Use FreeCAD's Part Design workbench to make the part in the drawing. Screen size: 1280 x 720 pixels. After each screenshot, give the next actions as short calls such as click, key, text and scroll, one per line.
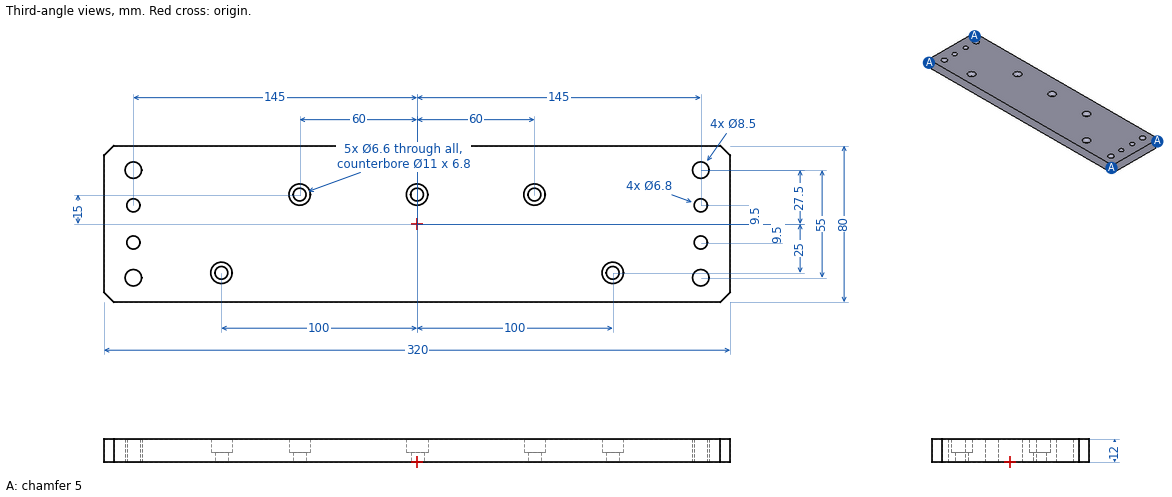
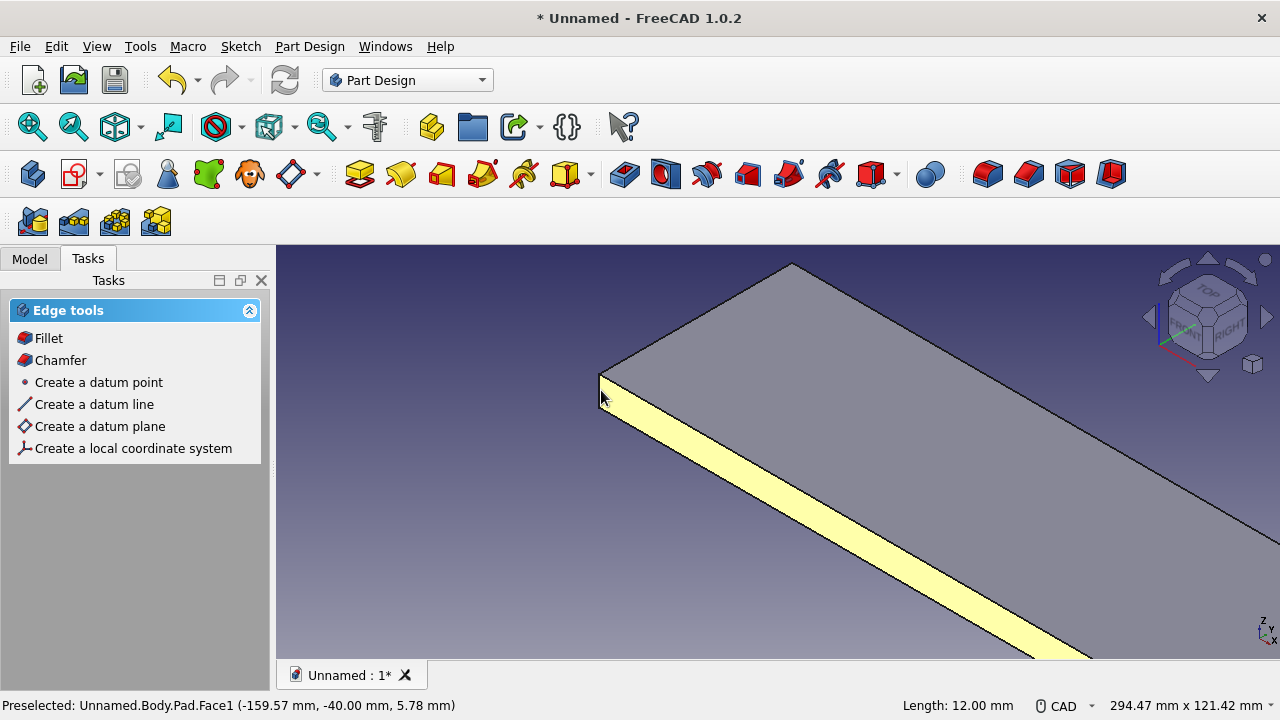
click(33, 128)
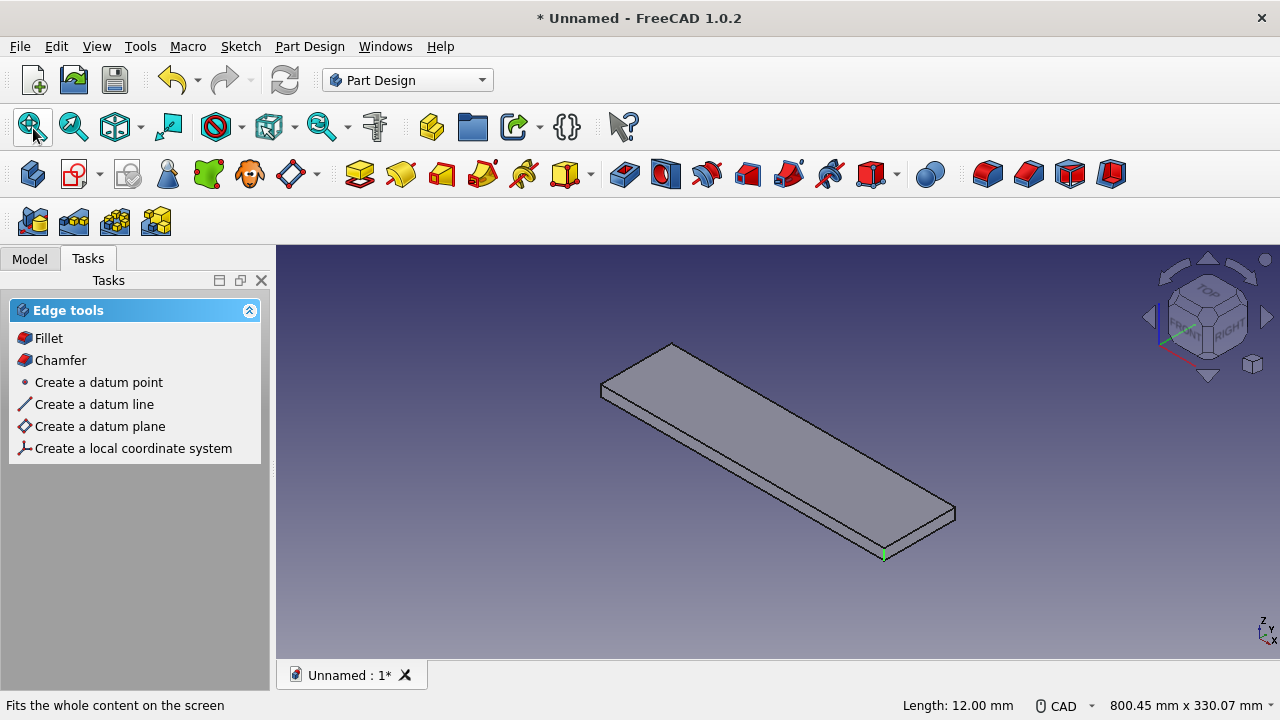
key(2)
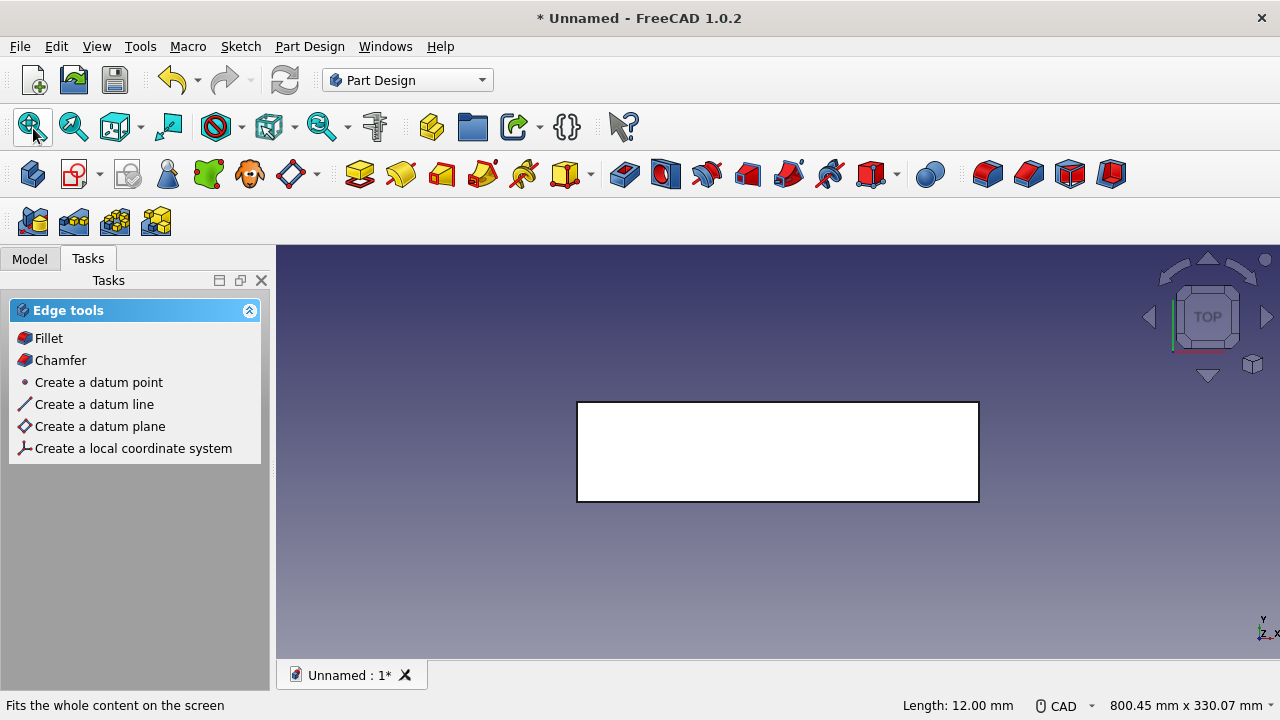
click(33, 128)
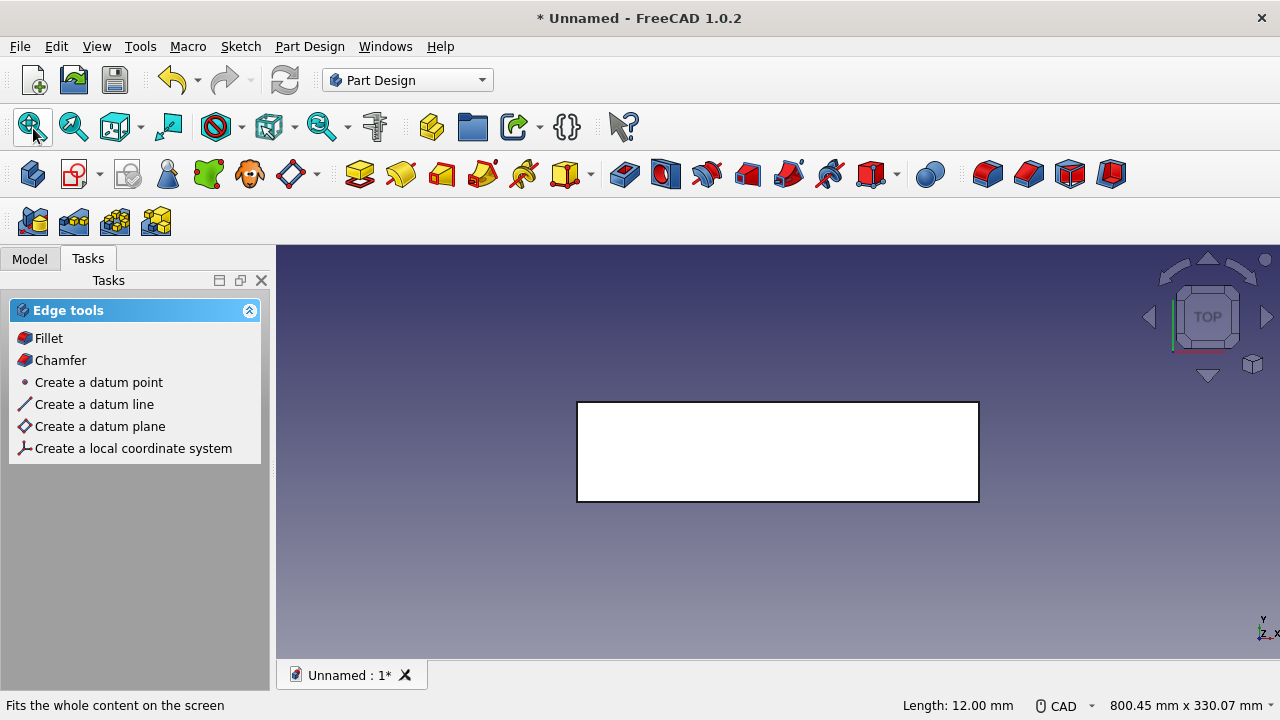
scroll(577, 501, up, 5)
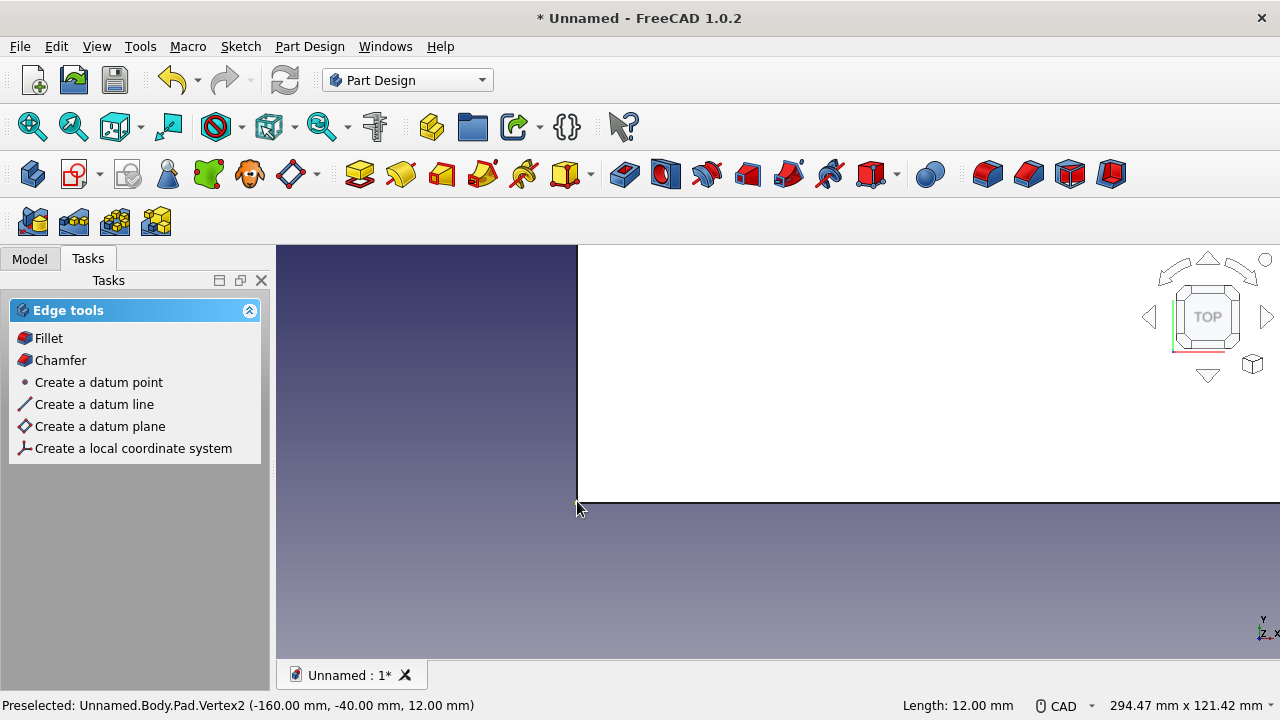
click(33, 128)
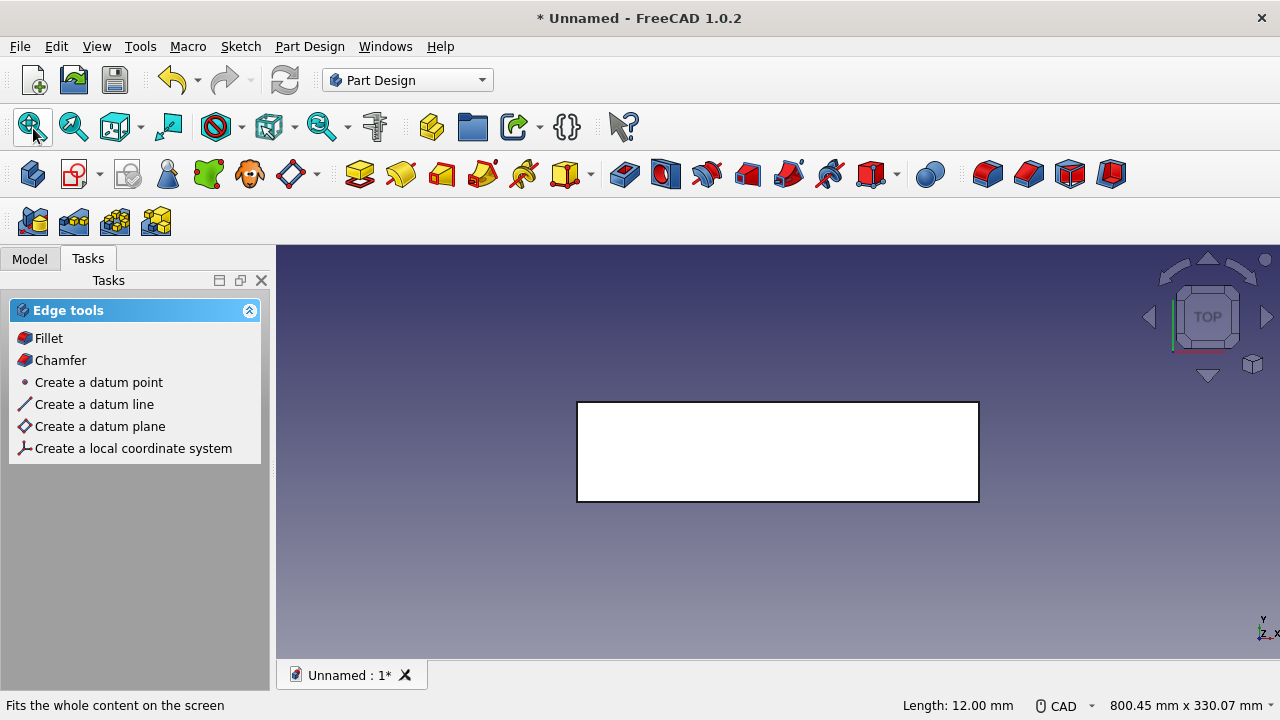
key(1)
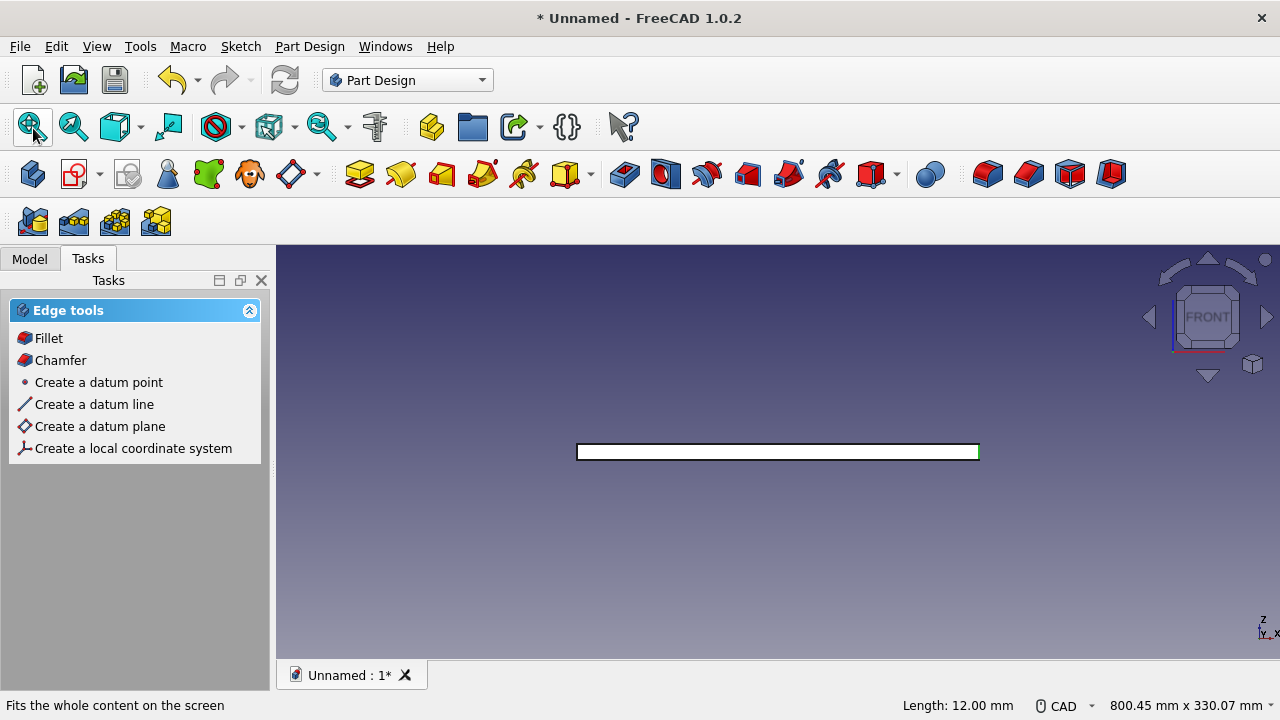
click(33, 128)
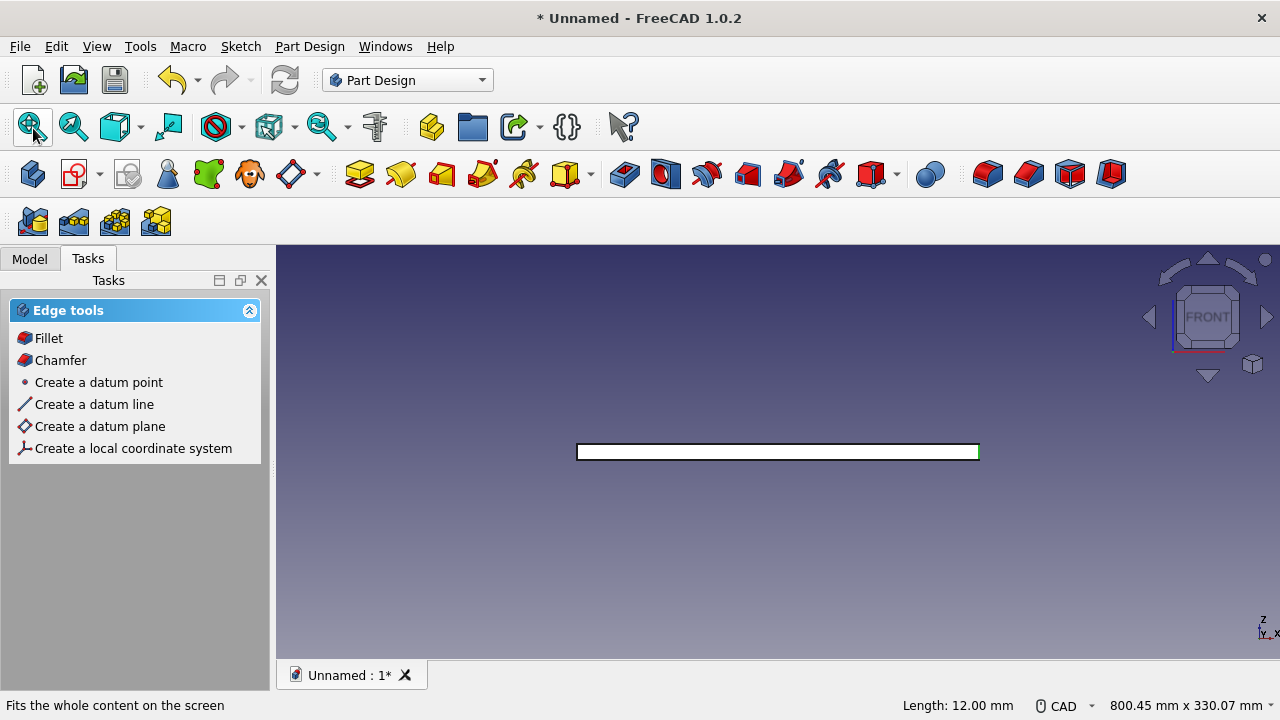
click(577, 451, ctrl)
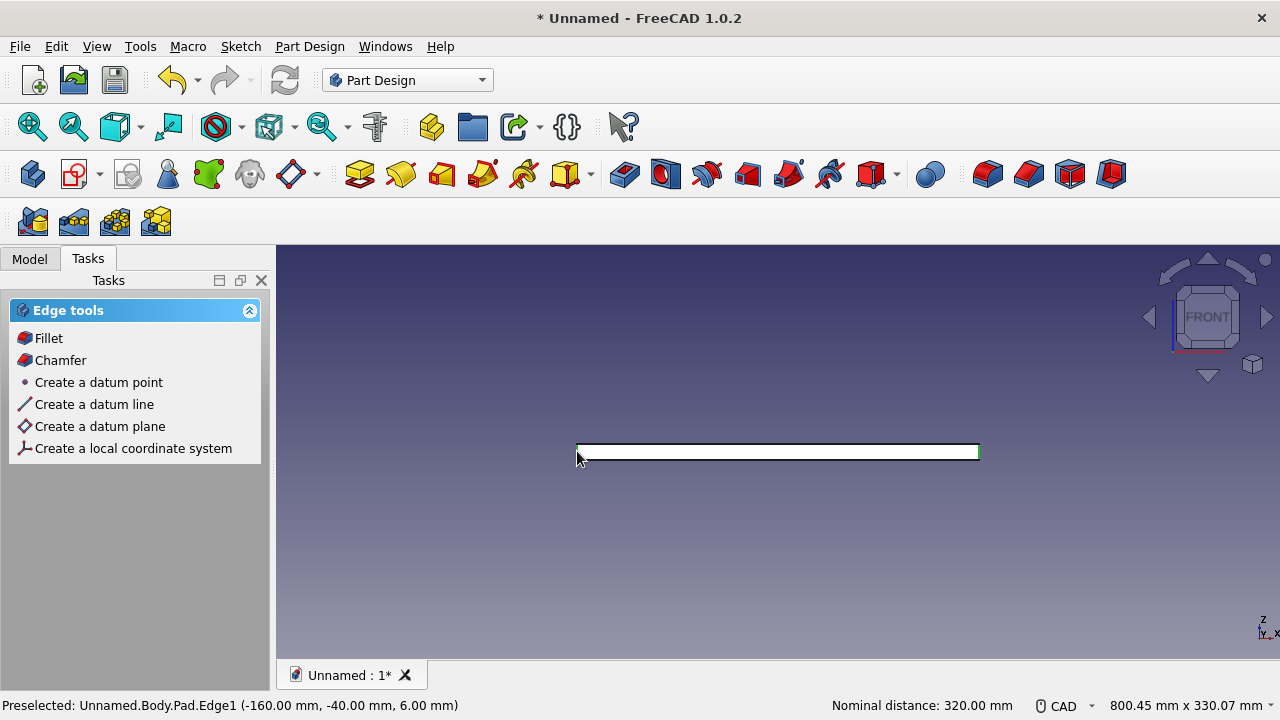
scroll(577, 451, up, 5)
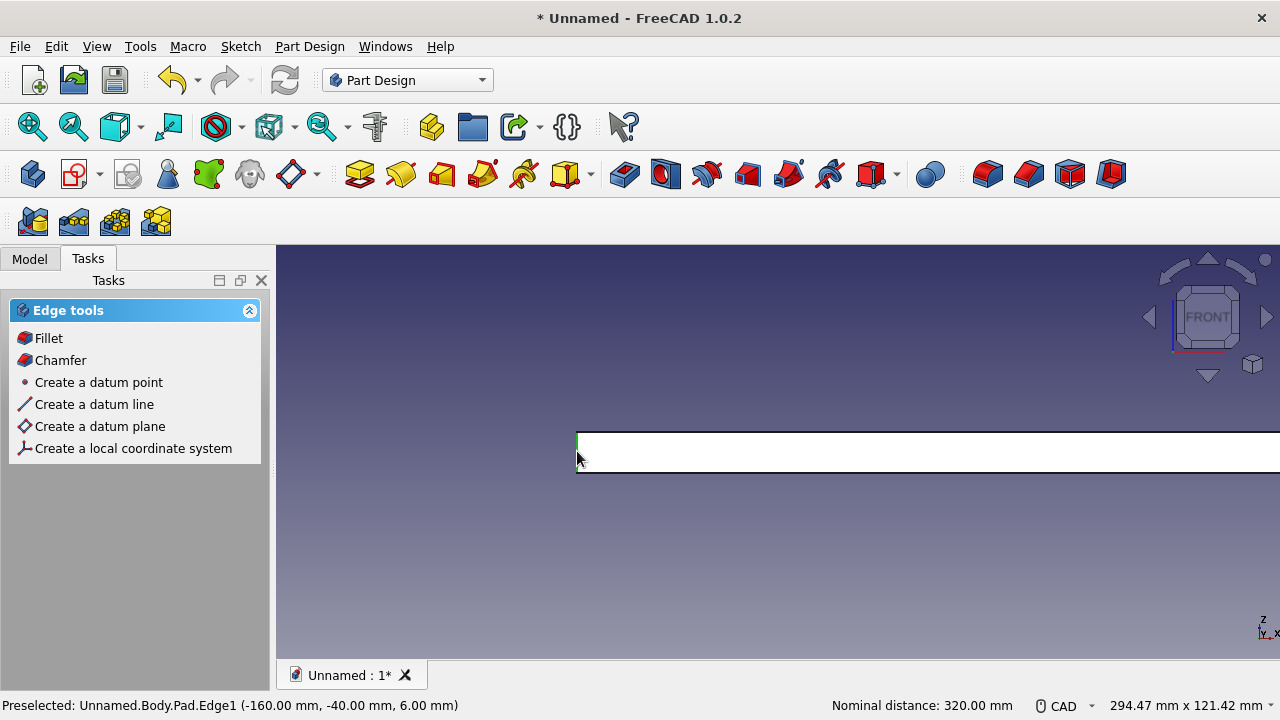
click(33, 128)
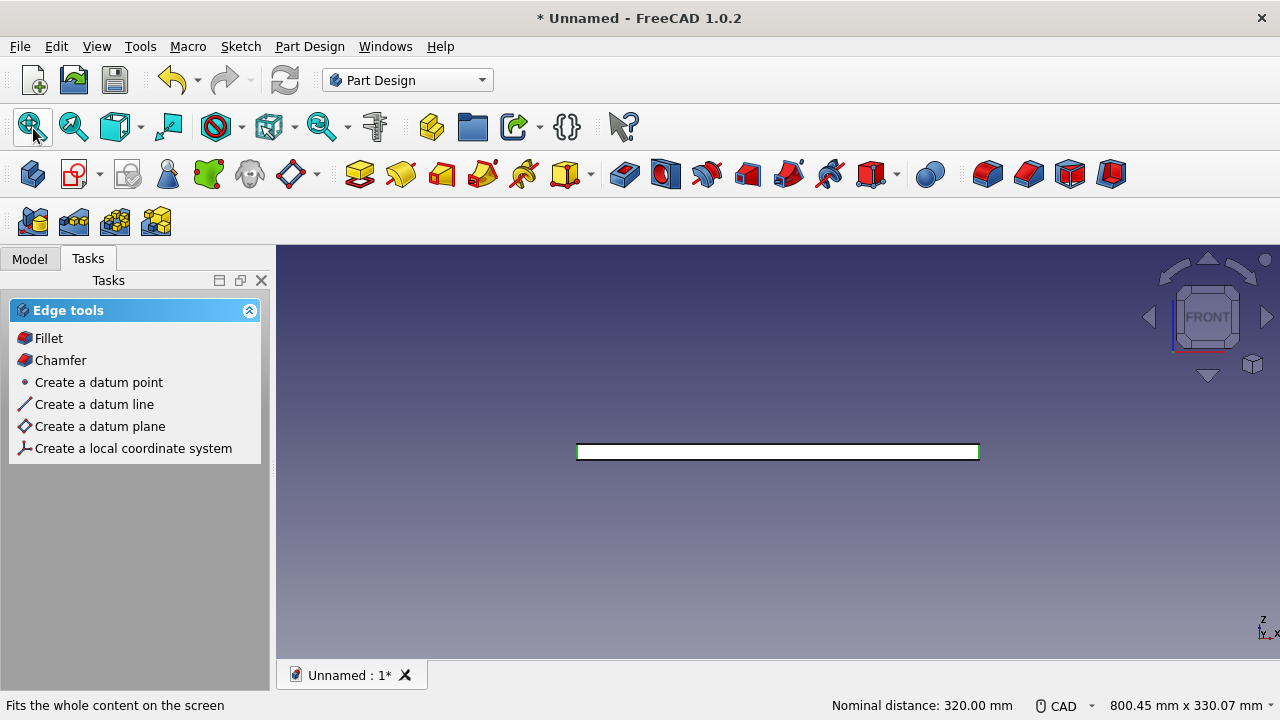
key(3)